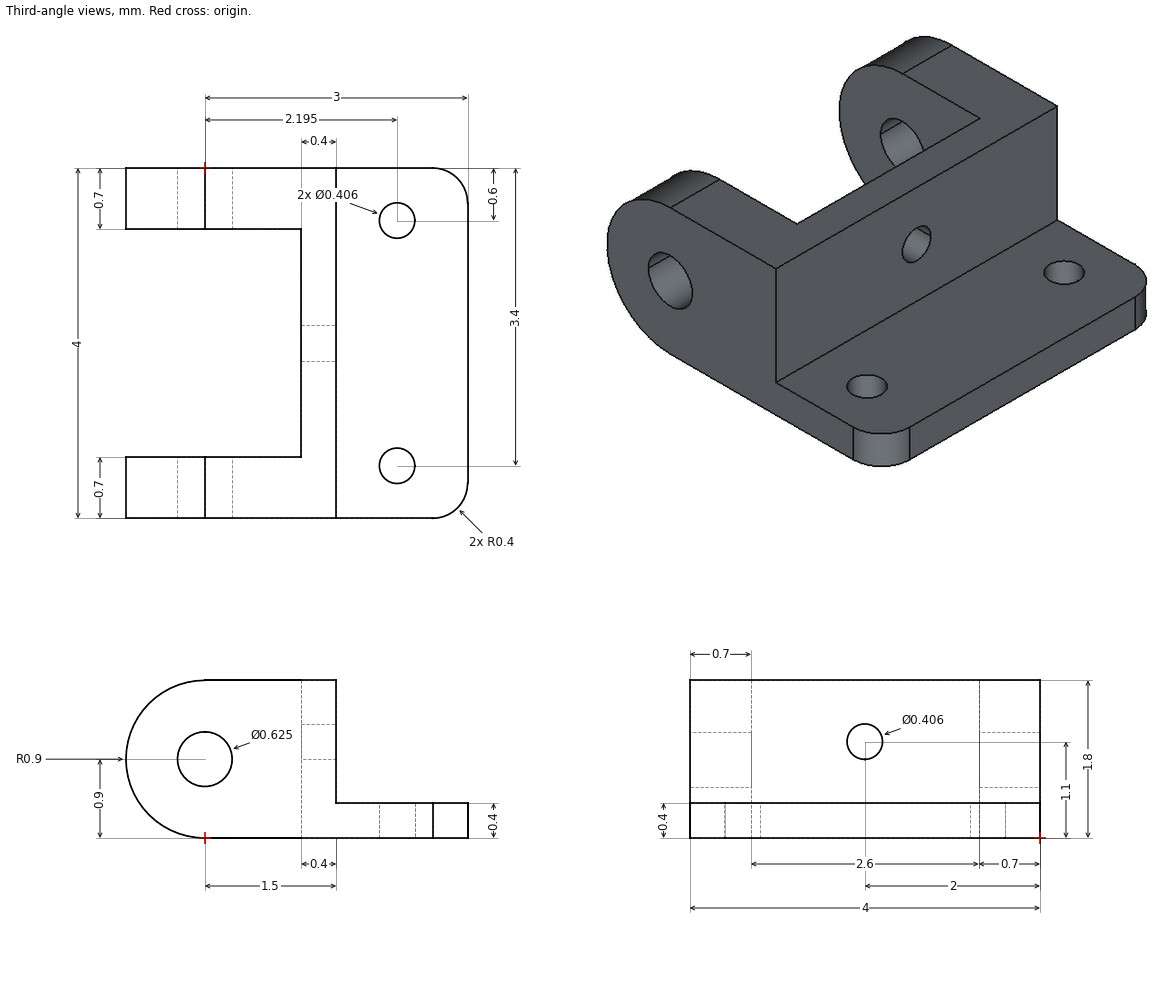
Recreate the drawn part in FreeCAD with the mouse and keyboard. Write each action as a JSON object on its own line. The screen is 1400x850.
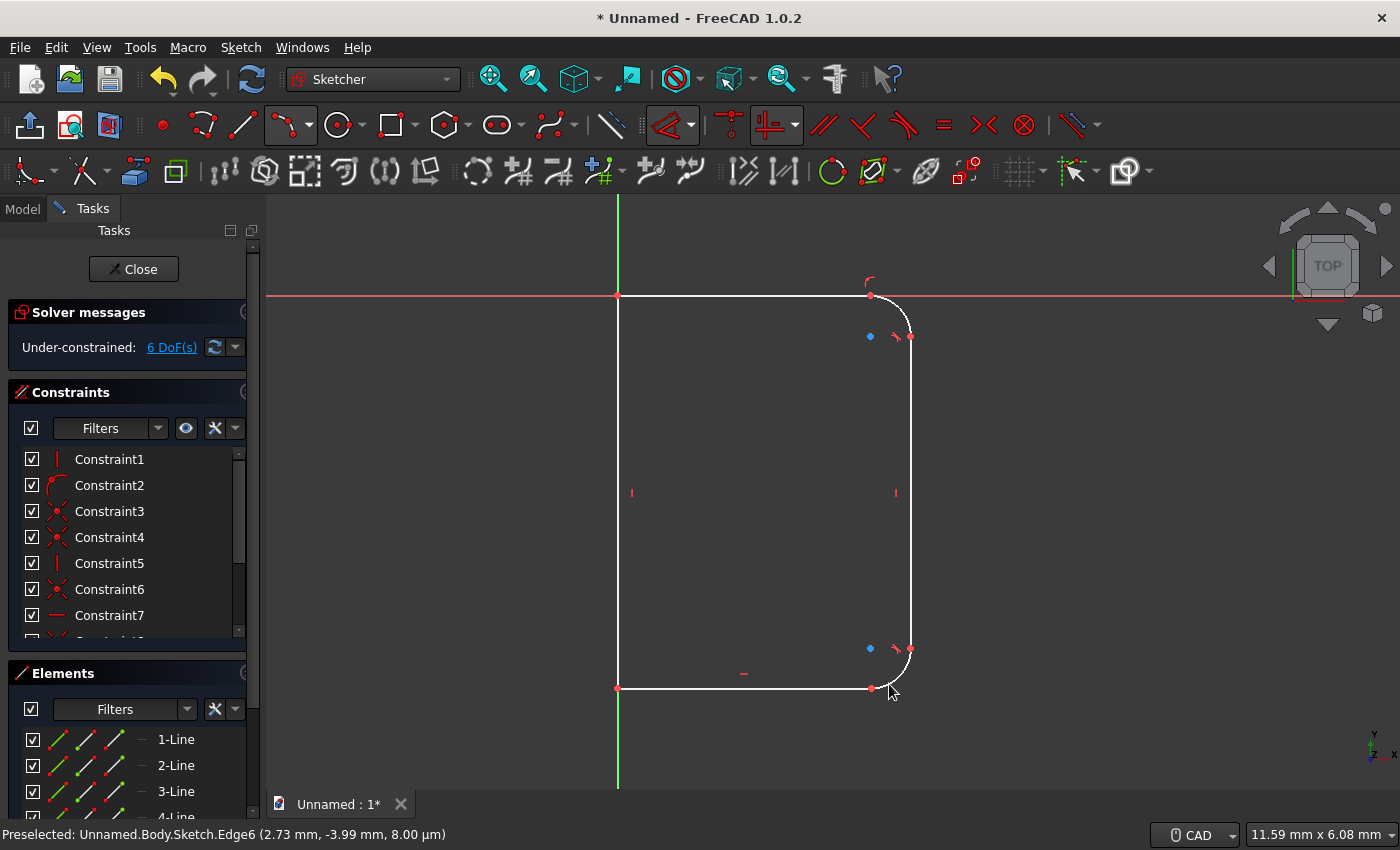
{"action": "left_click", "coordinate": [795, 296]}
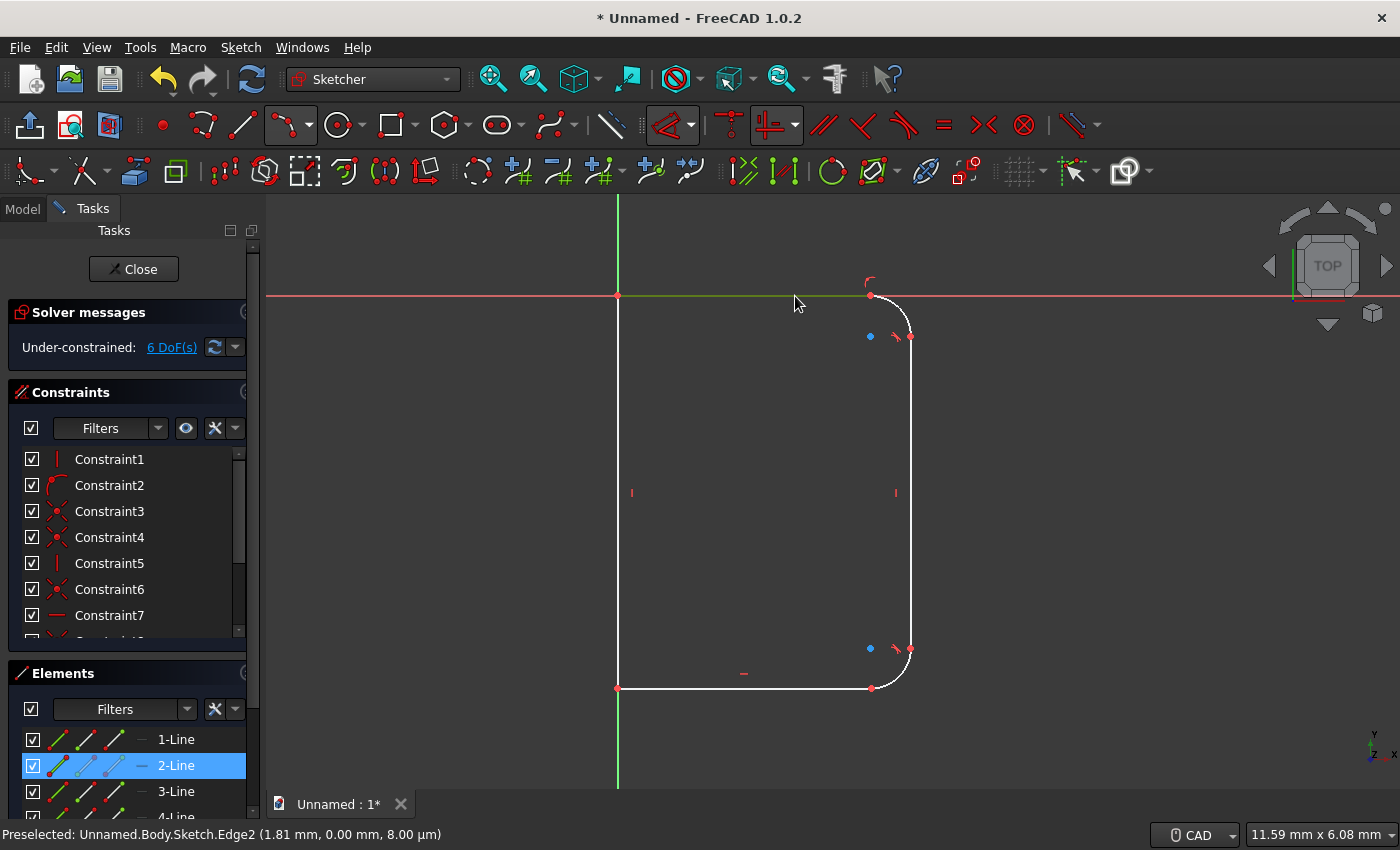
{"action": "left_click", "coordinate": [907, 318]}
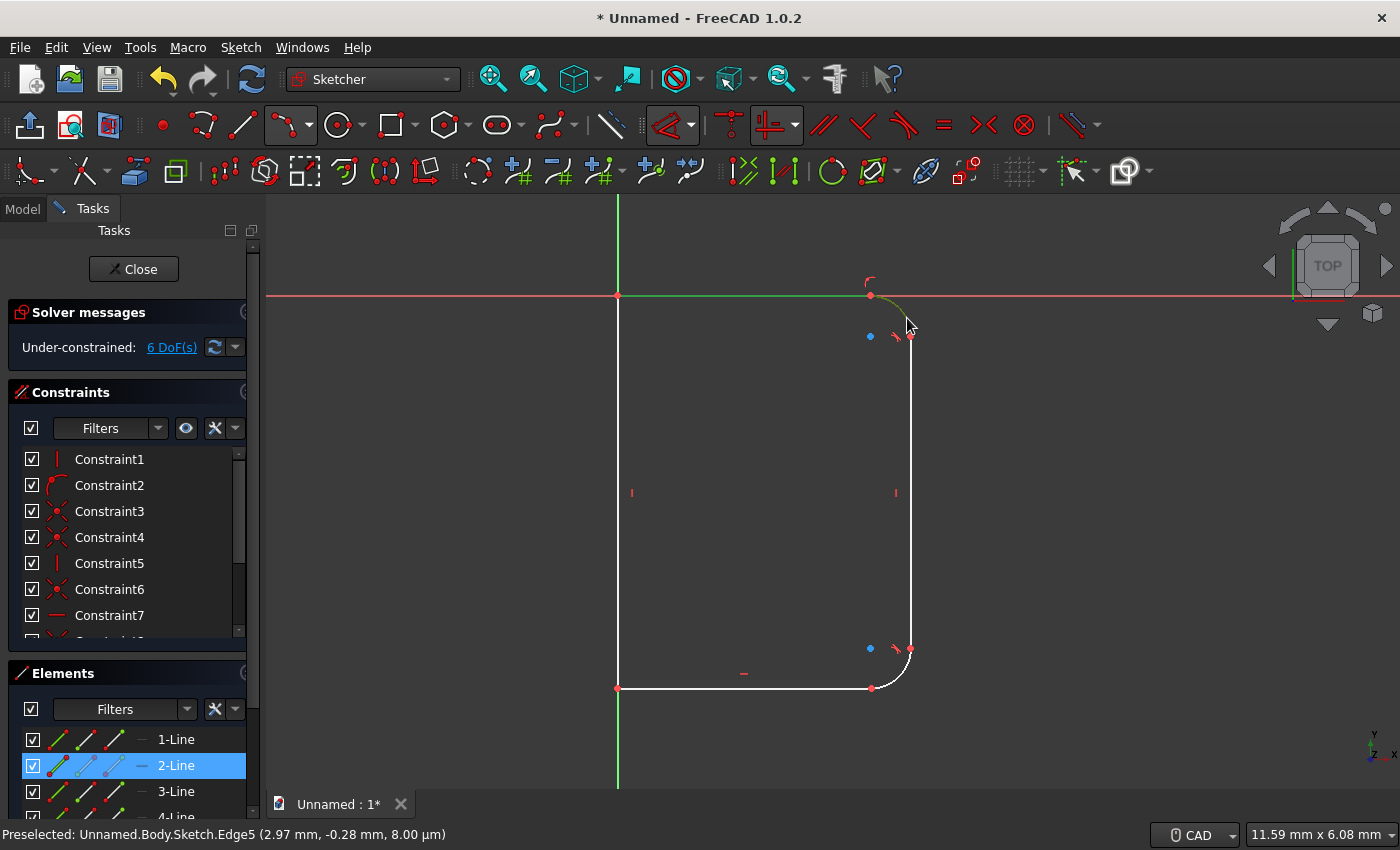
{"action": "key", "text": "t"}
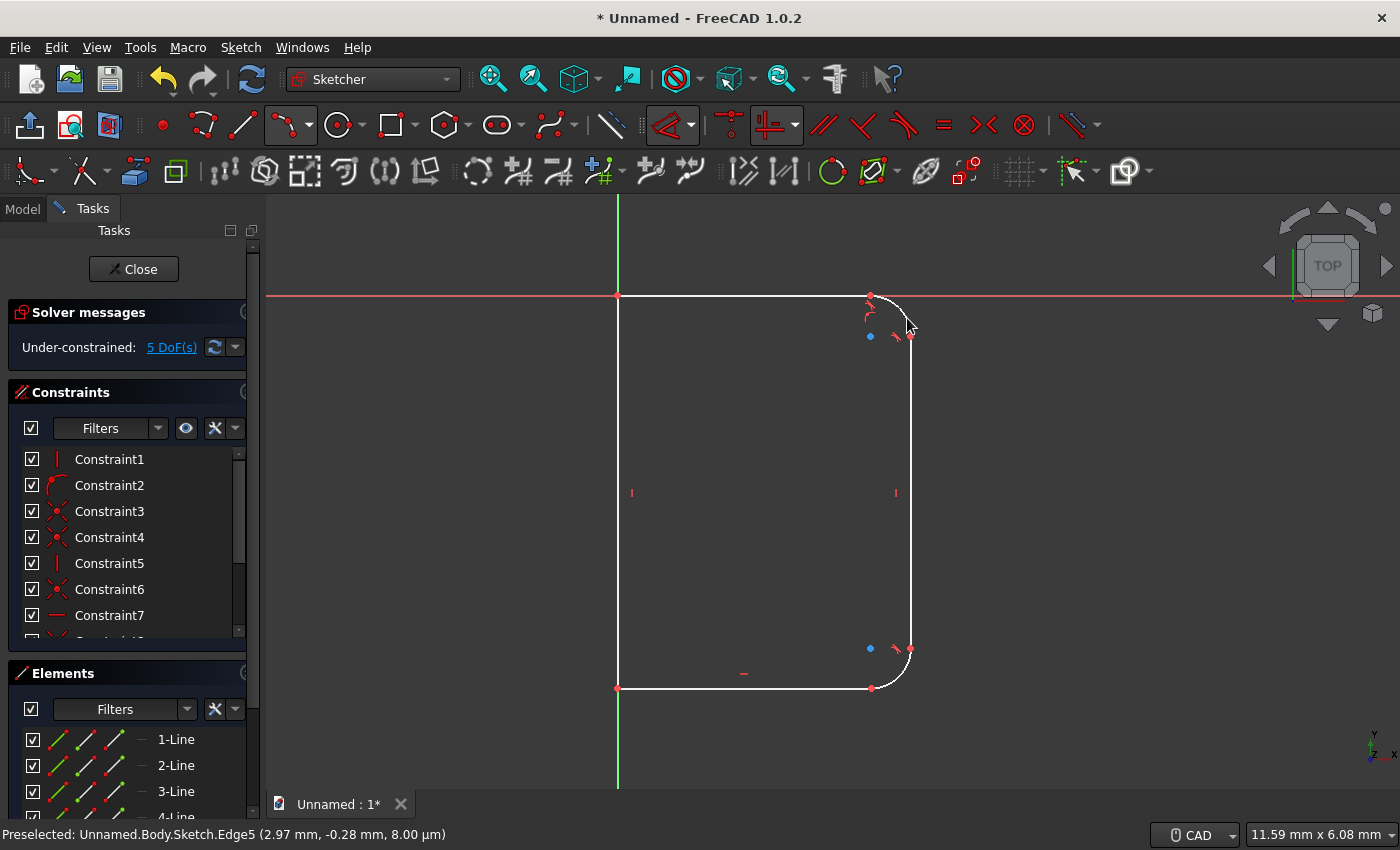
{"action": "left_click", "coordinate": [694, 689]}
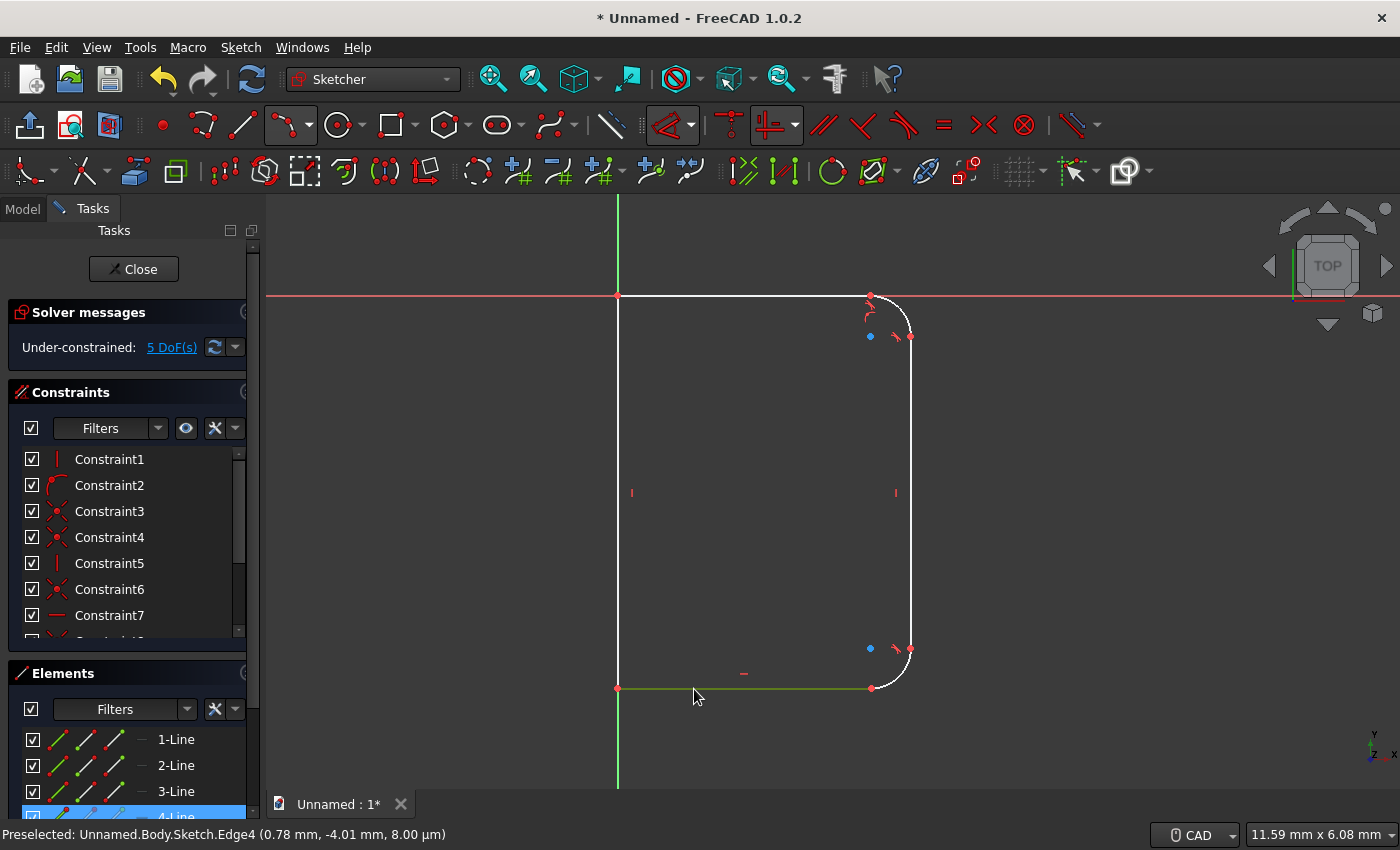
{"action": "left_click", "coordinate": [890, 684]}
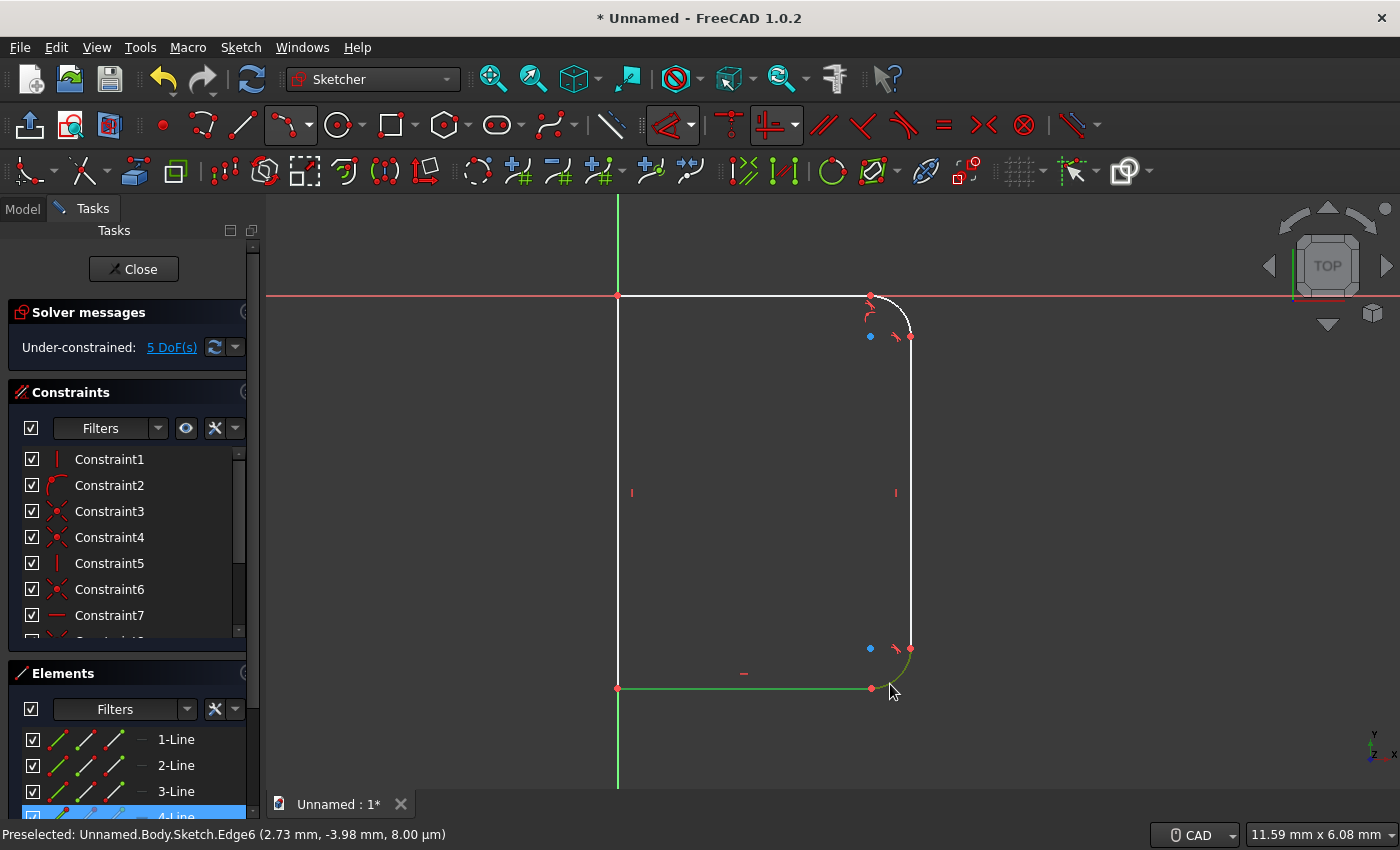
{"action": "key", "text": "t"}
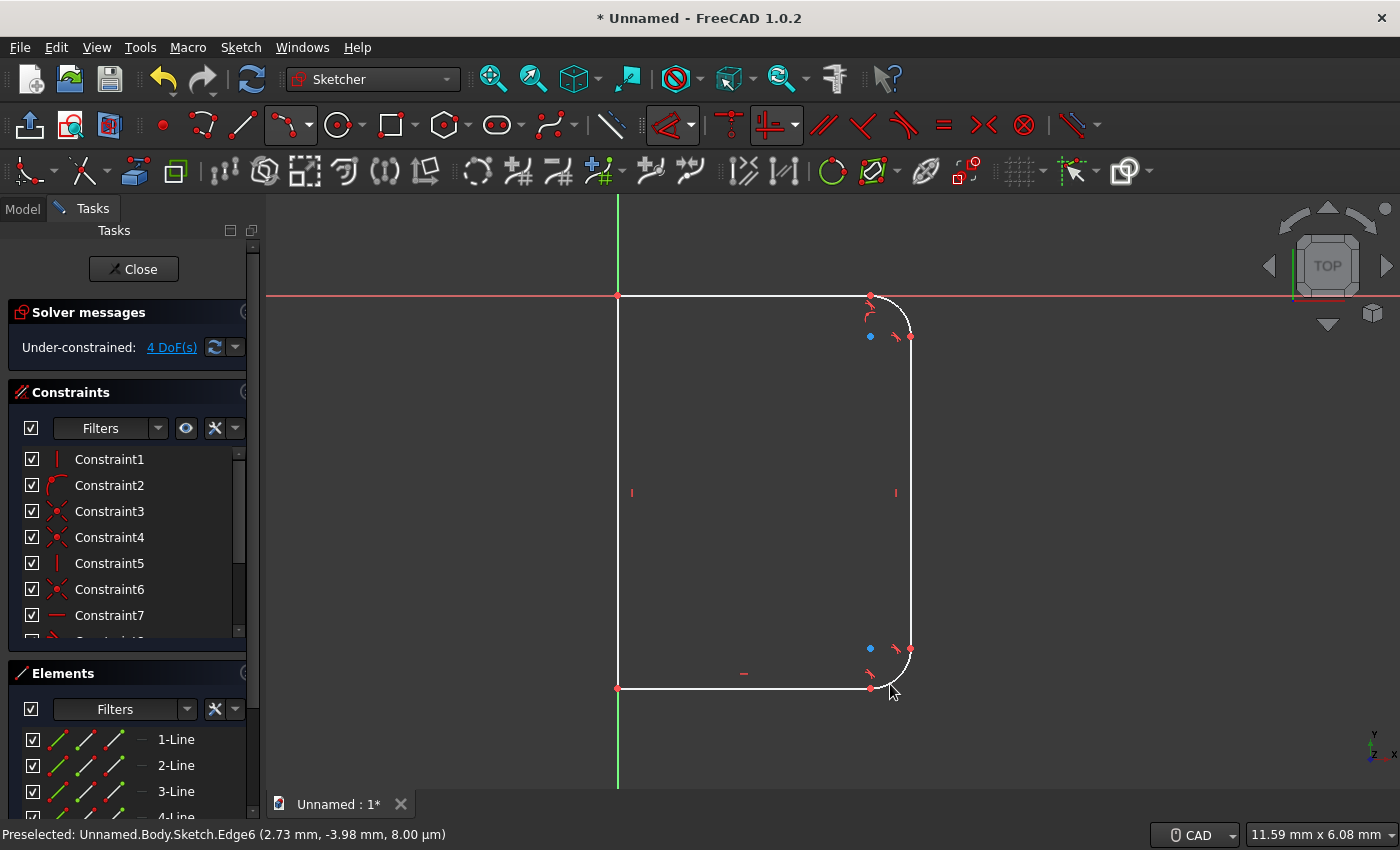
{"action": "left_click", "coordinate": [907, 318]}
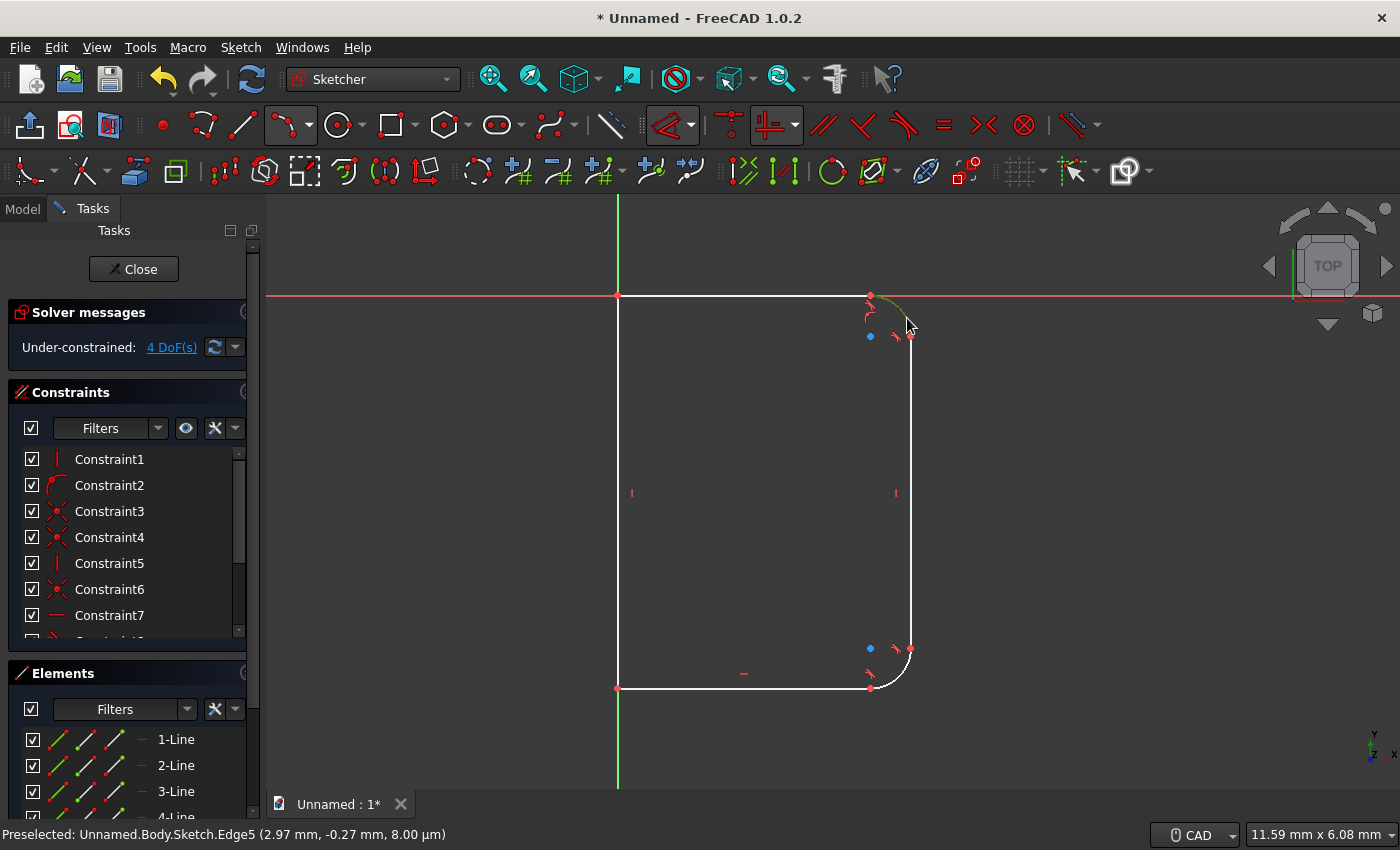
{"action": "left_click", "coordinate": [889, 684]}